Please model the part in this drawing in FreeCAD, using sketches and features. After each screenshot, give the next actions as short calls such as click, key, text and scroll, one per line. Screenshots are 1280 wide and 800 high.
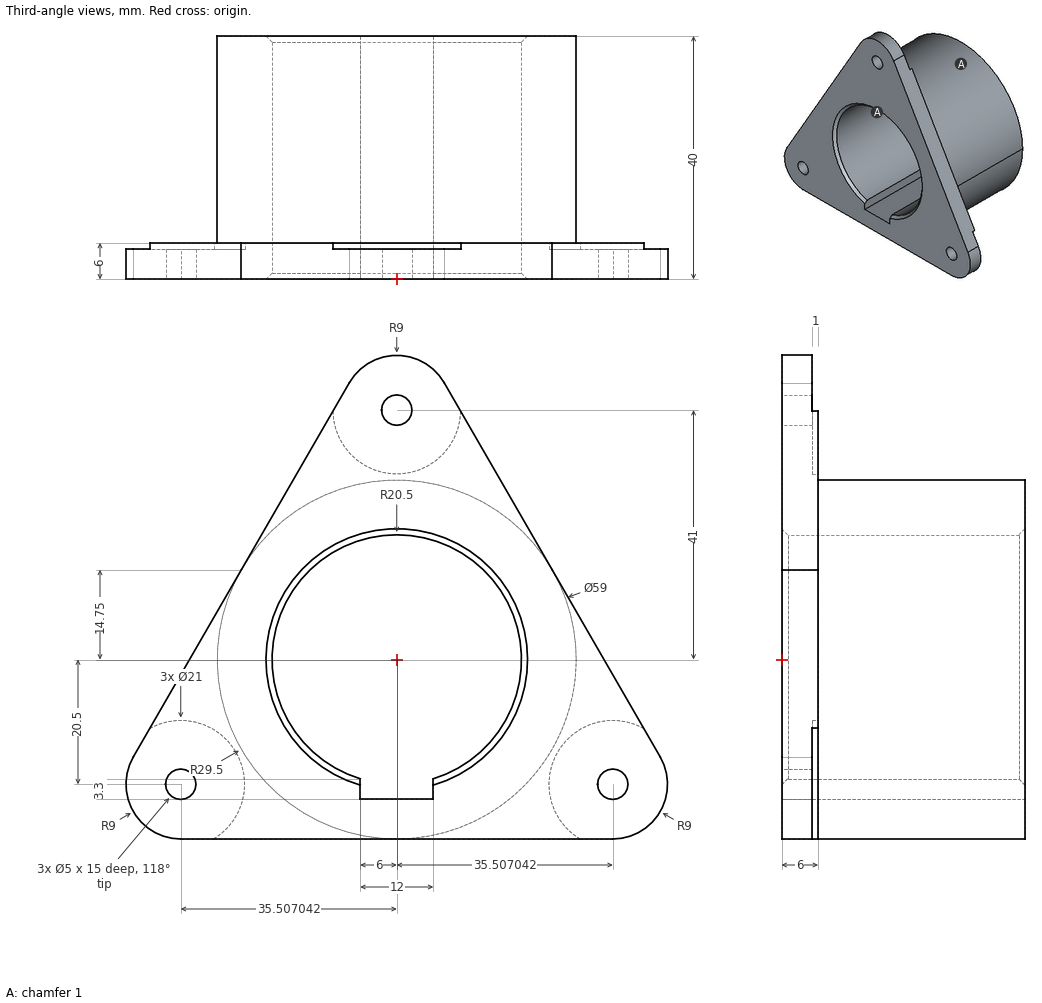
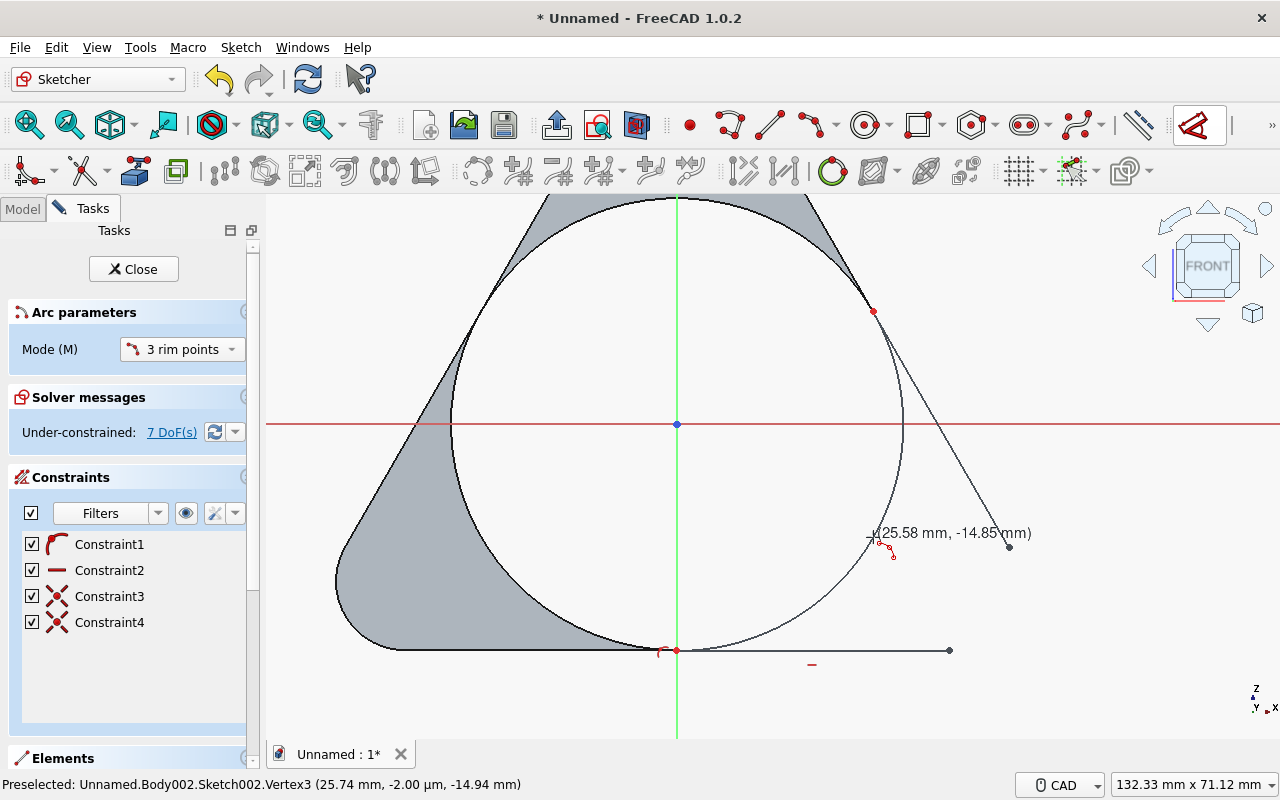
click(1009, 548)
click(949, 651)
click(1009, 616)
key(Escape)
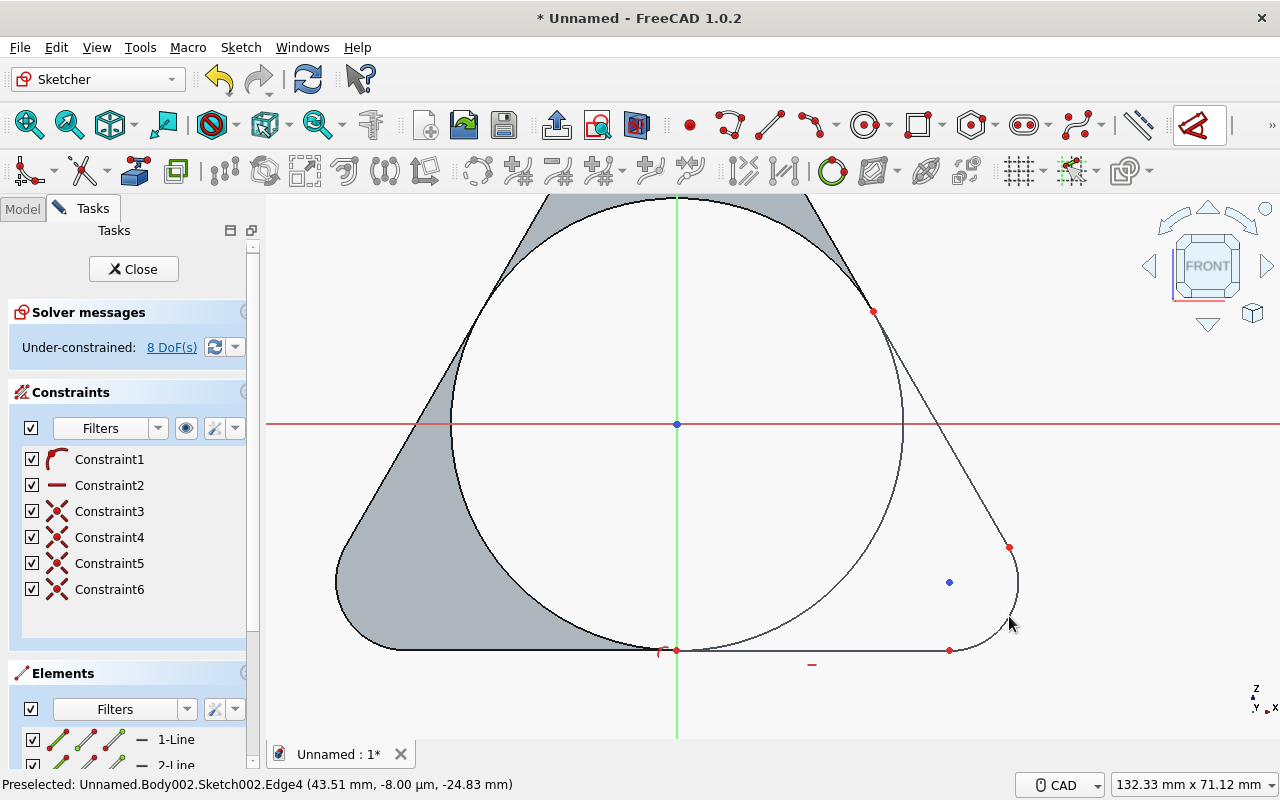
click(867, 651)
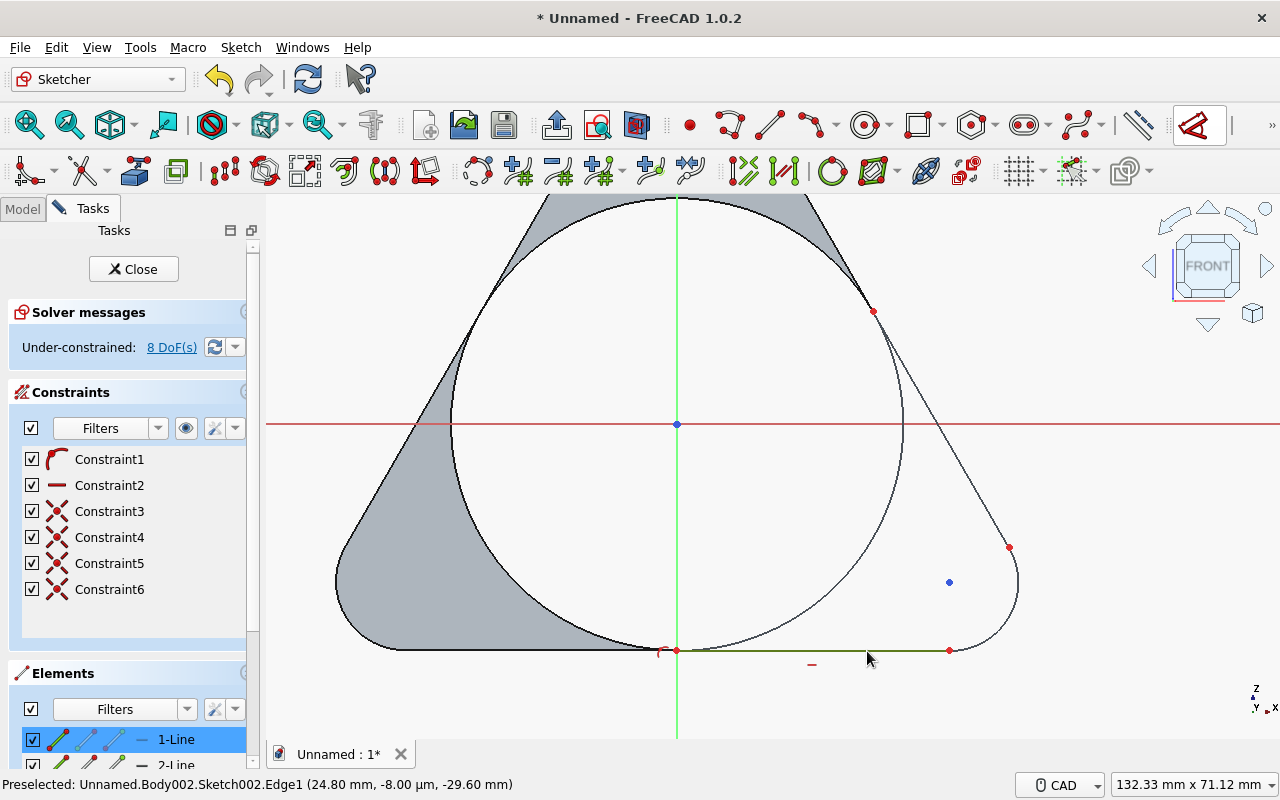
click(810, 608)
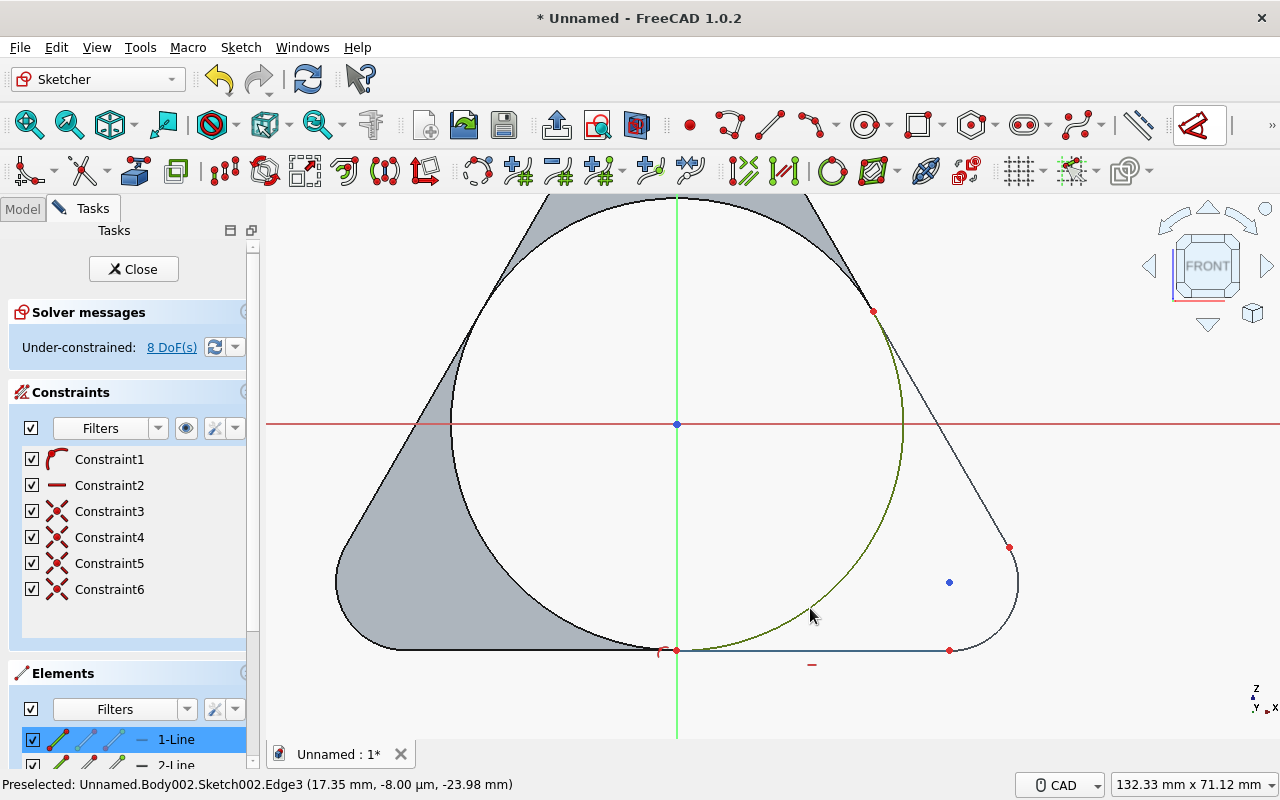
key(t)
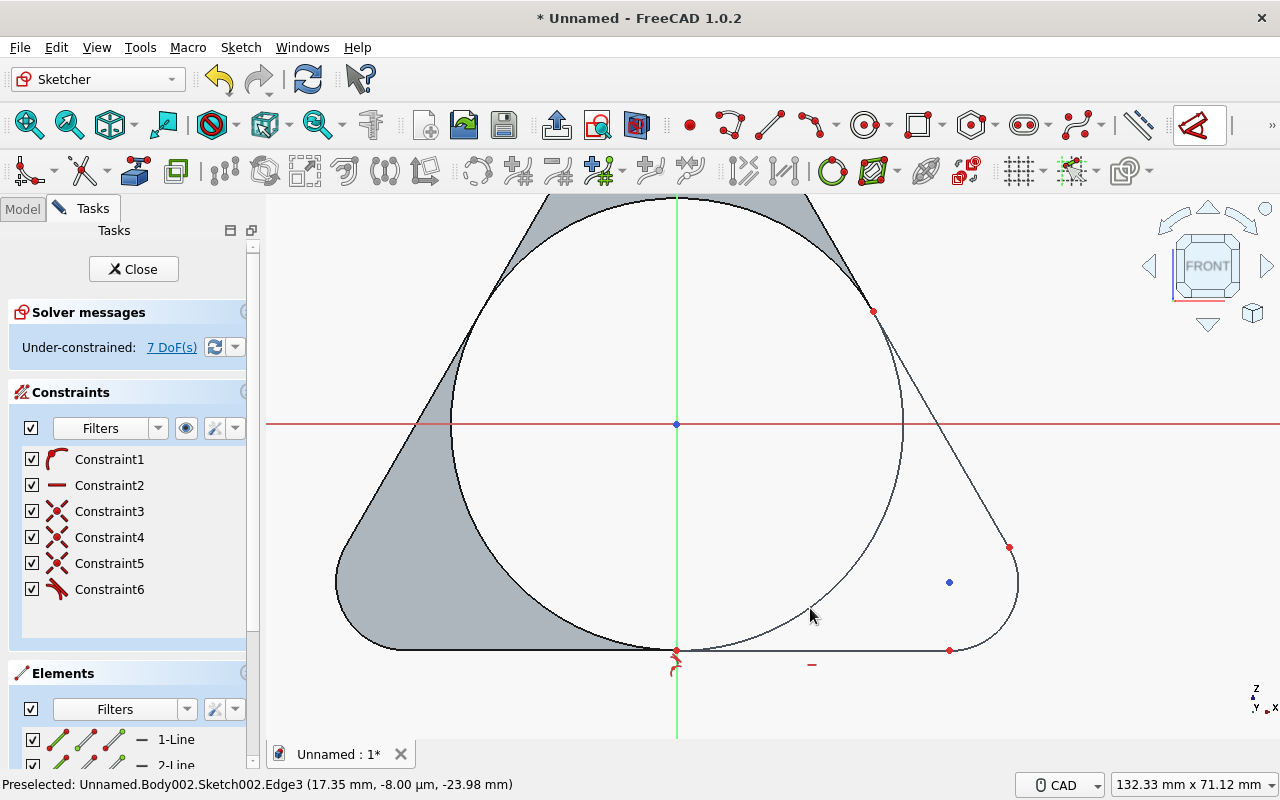
click(867, 651)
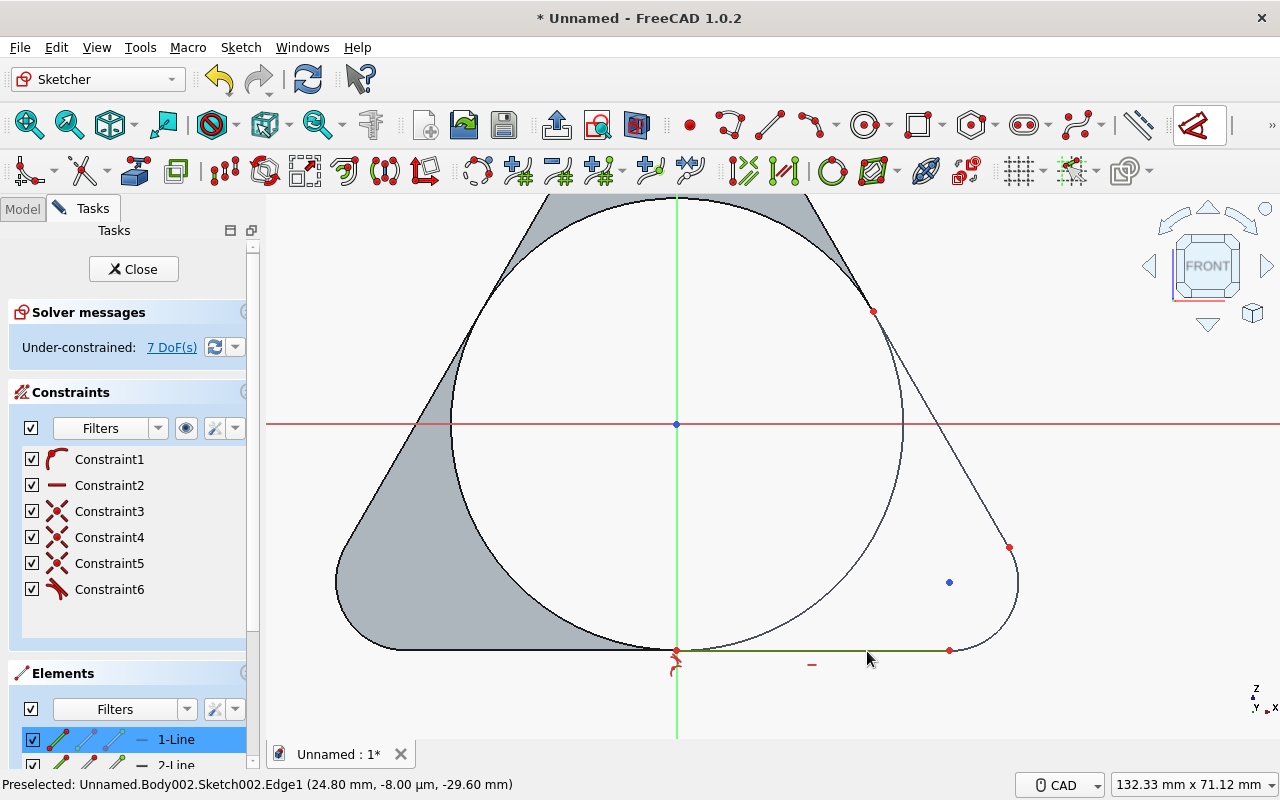
click(990, 638)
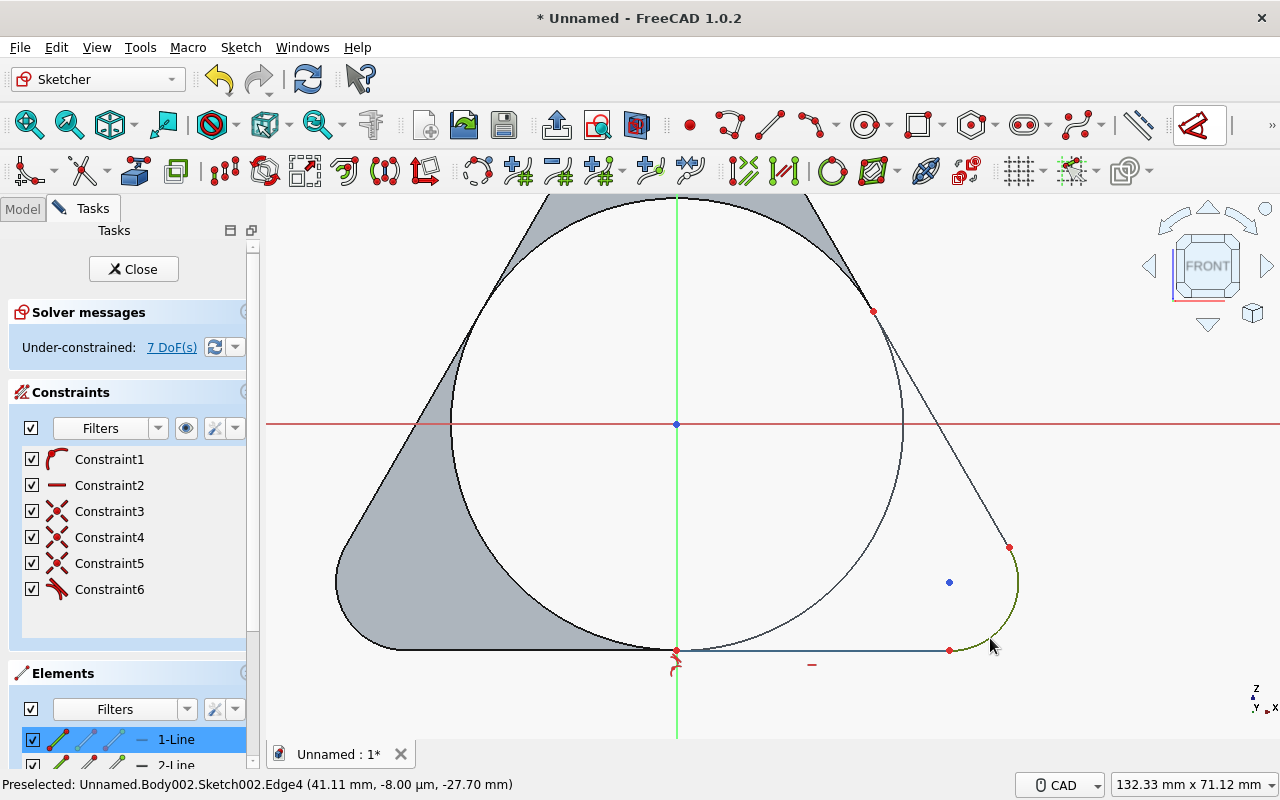
key(t)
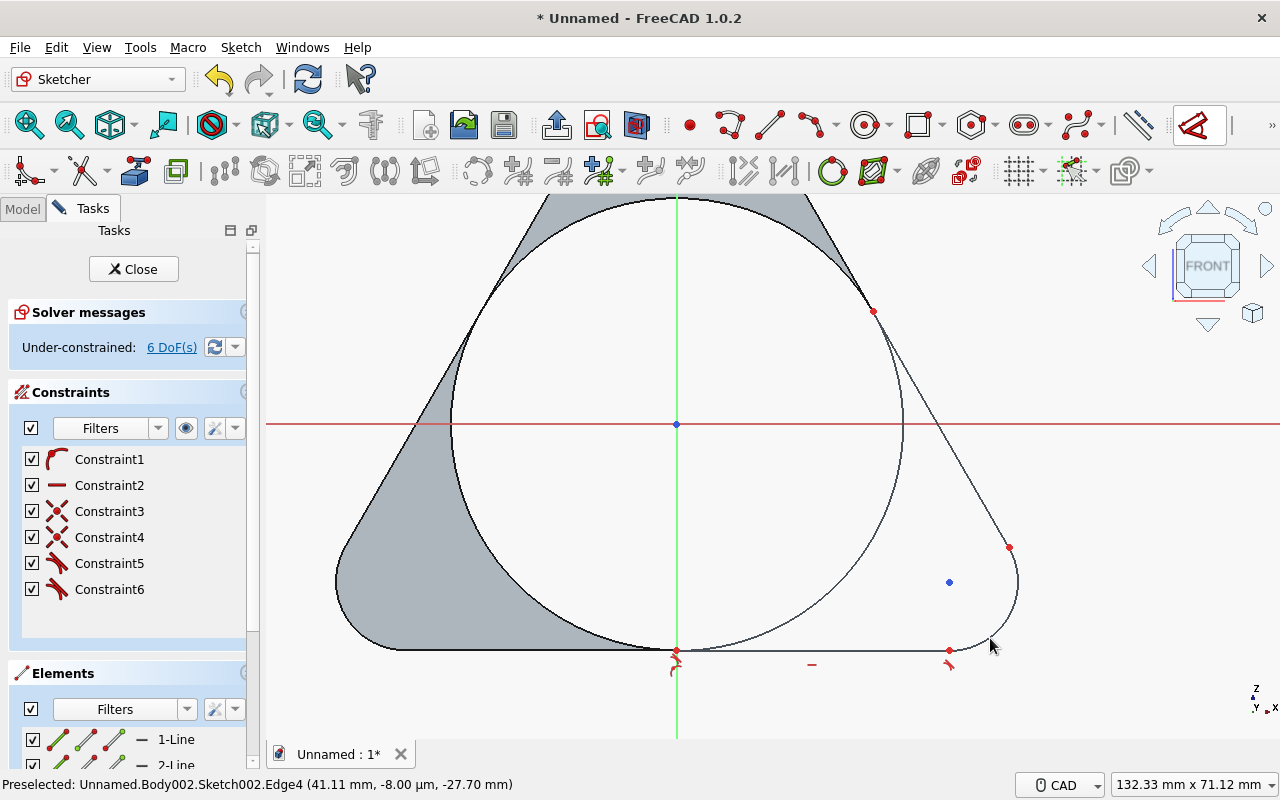
click(914, 383)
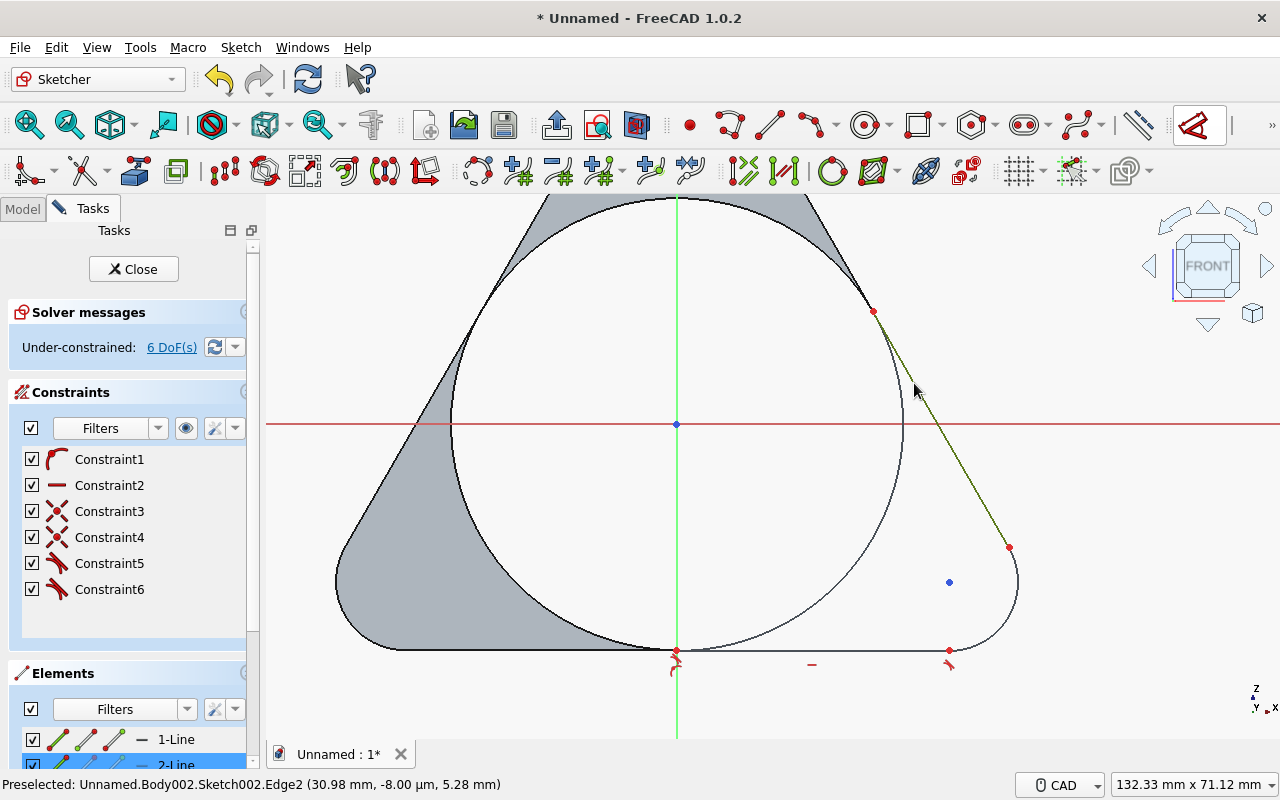
click(810, 608)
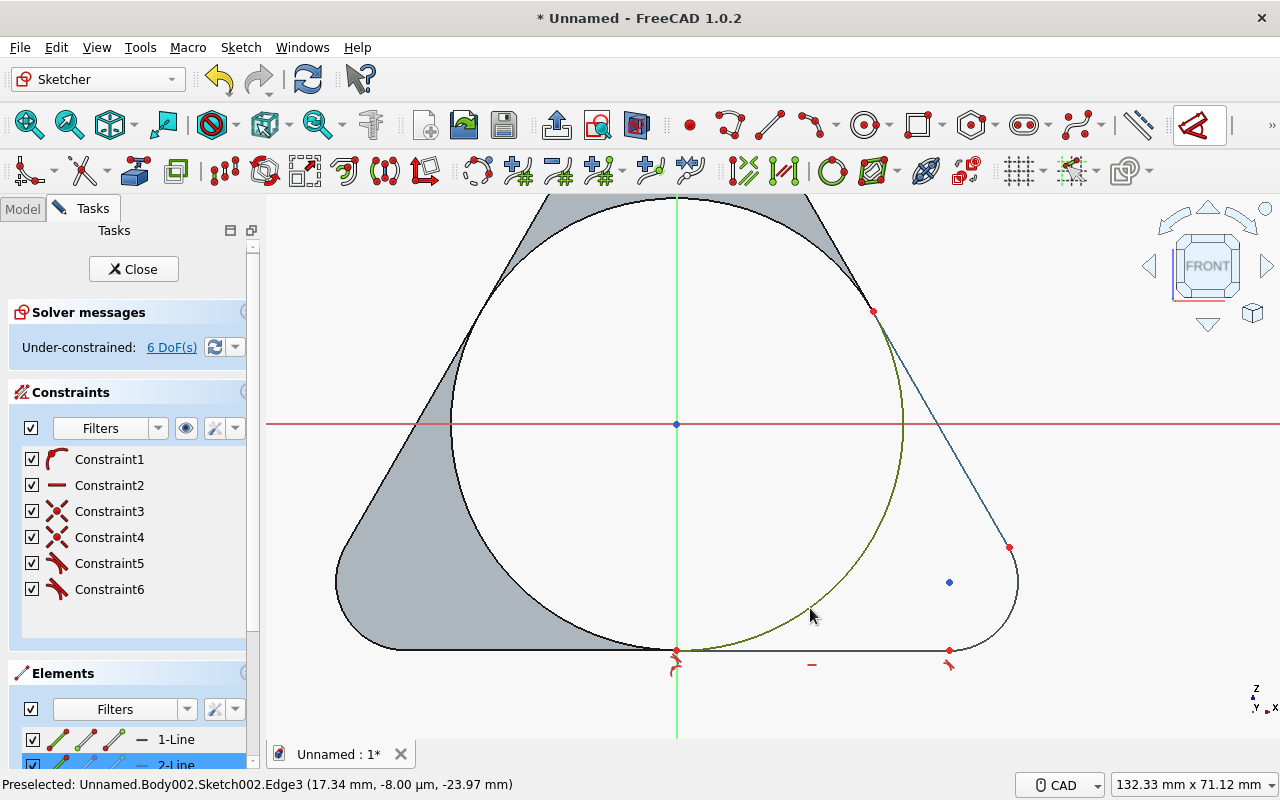
key(t)